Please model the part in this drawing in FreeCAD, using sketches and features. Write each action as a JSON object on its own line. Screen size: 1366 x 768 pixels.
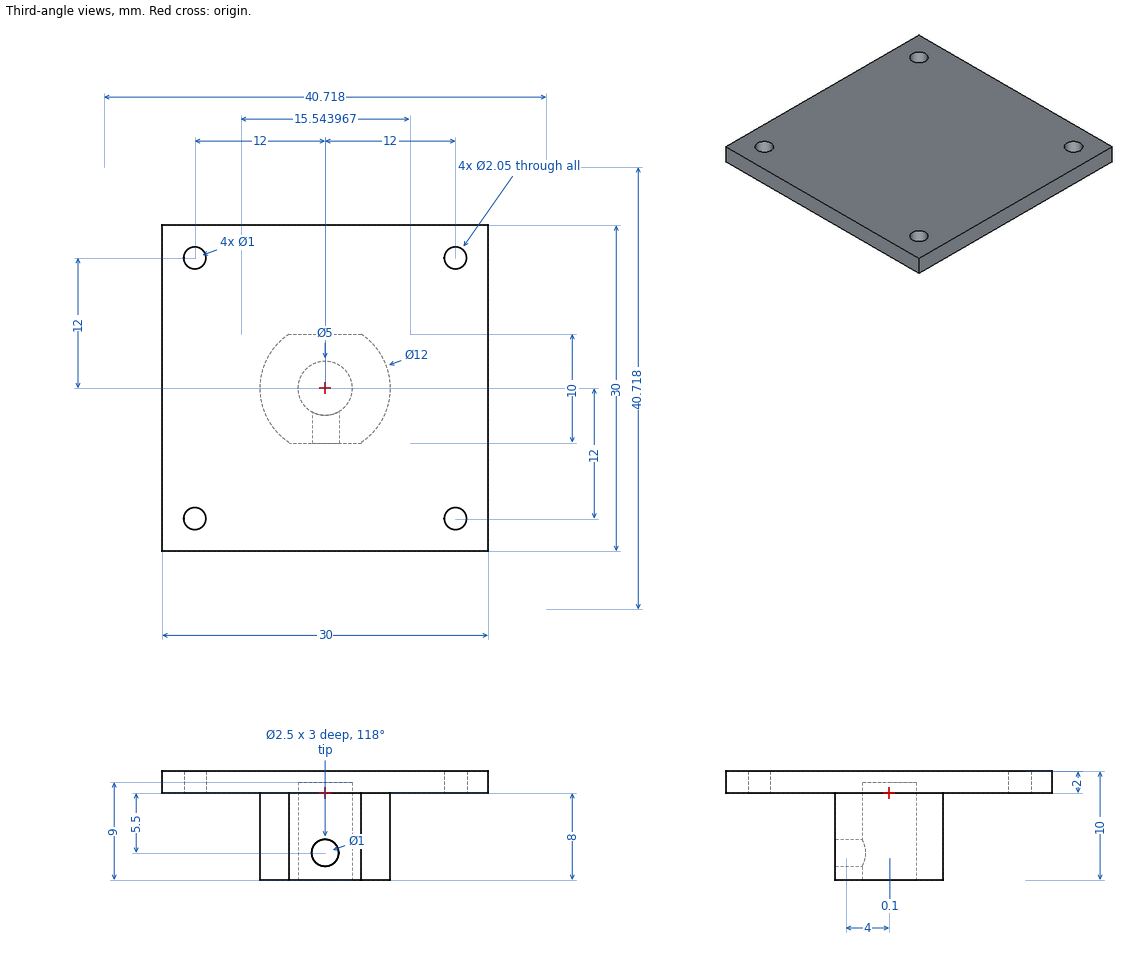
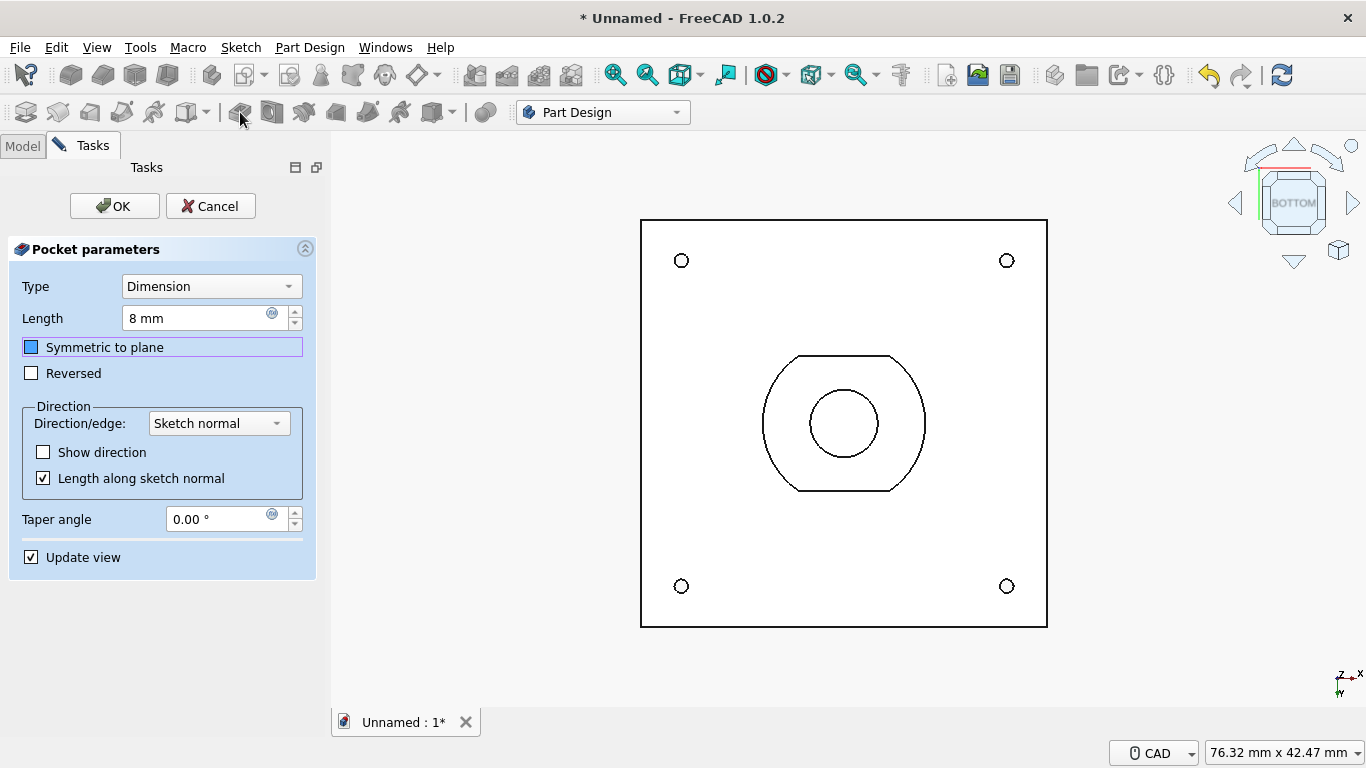
{"action": "left_click", "coordinate": [115, 206]}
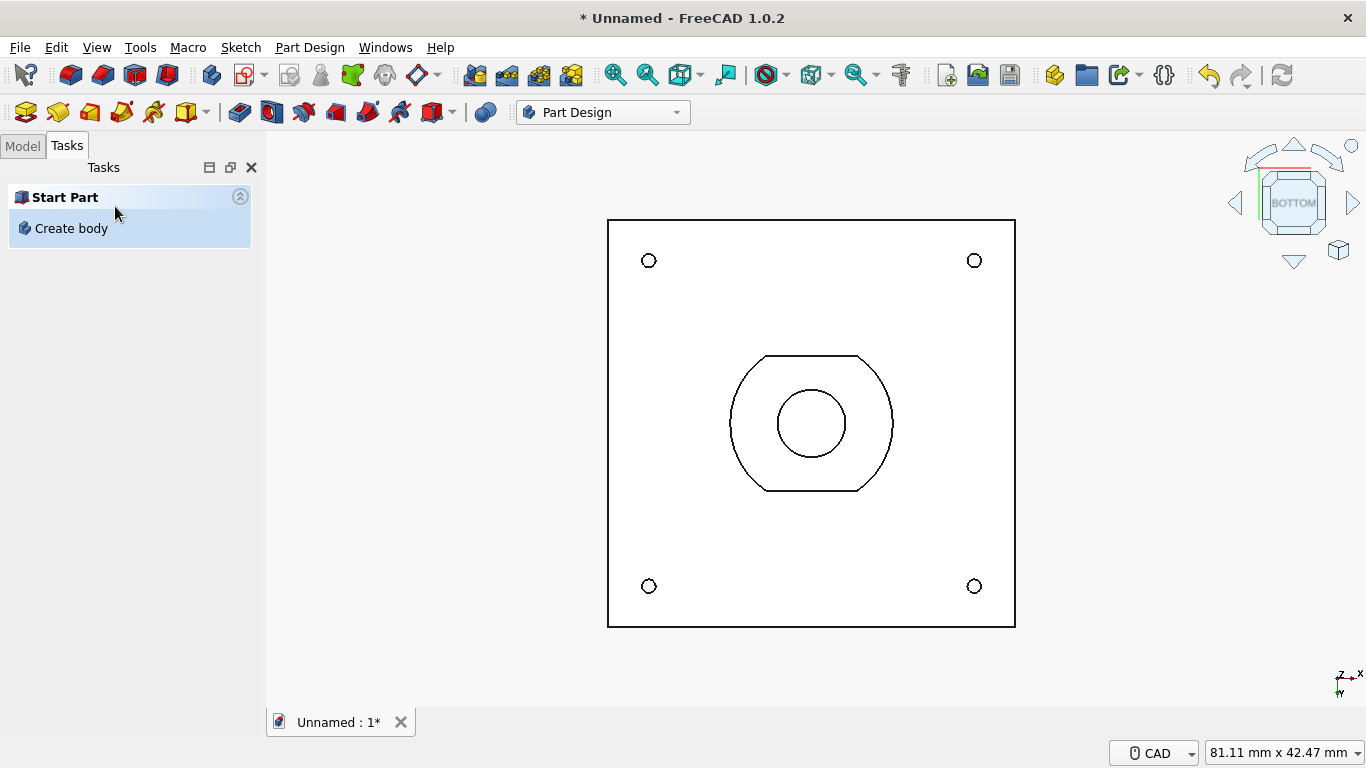
{"action": "key", "text": "0"}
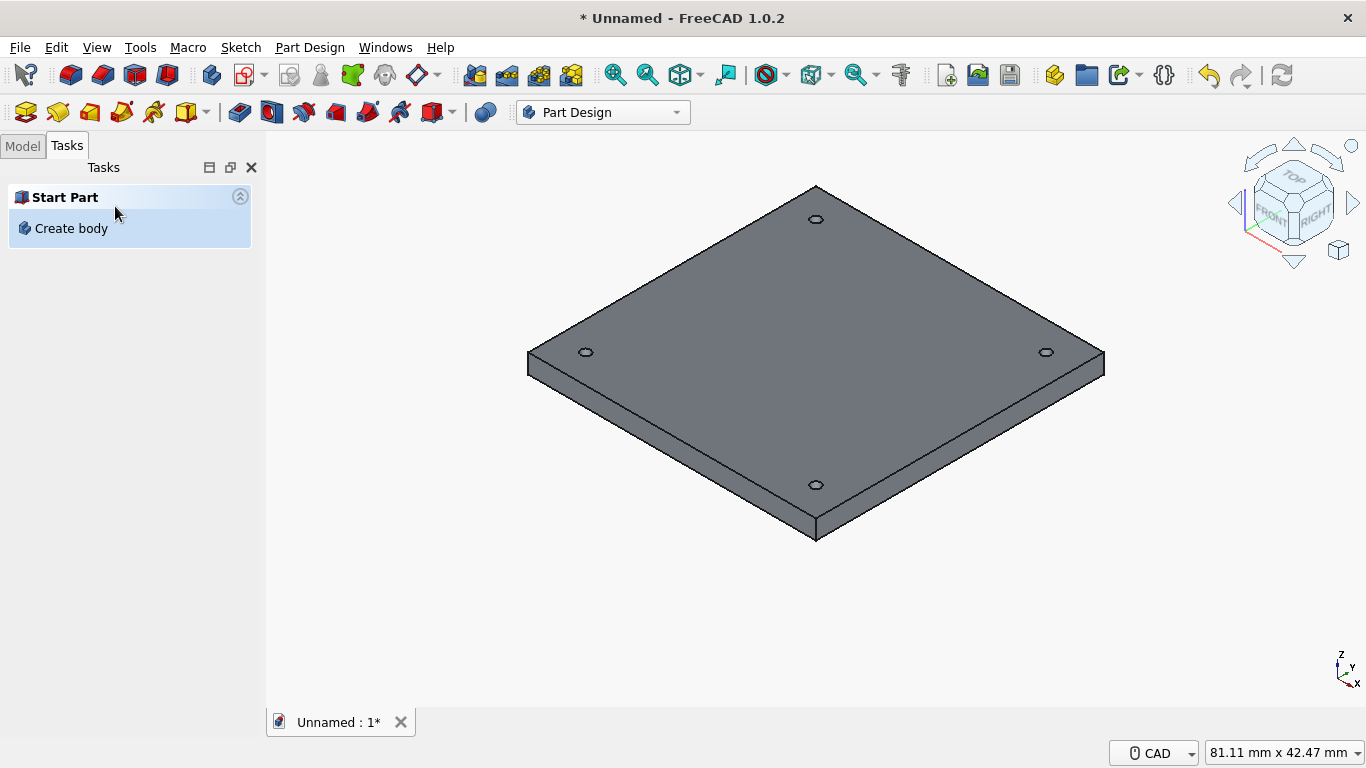
{"action": "key", "text": "1"}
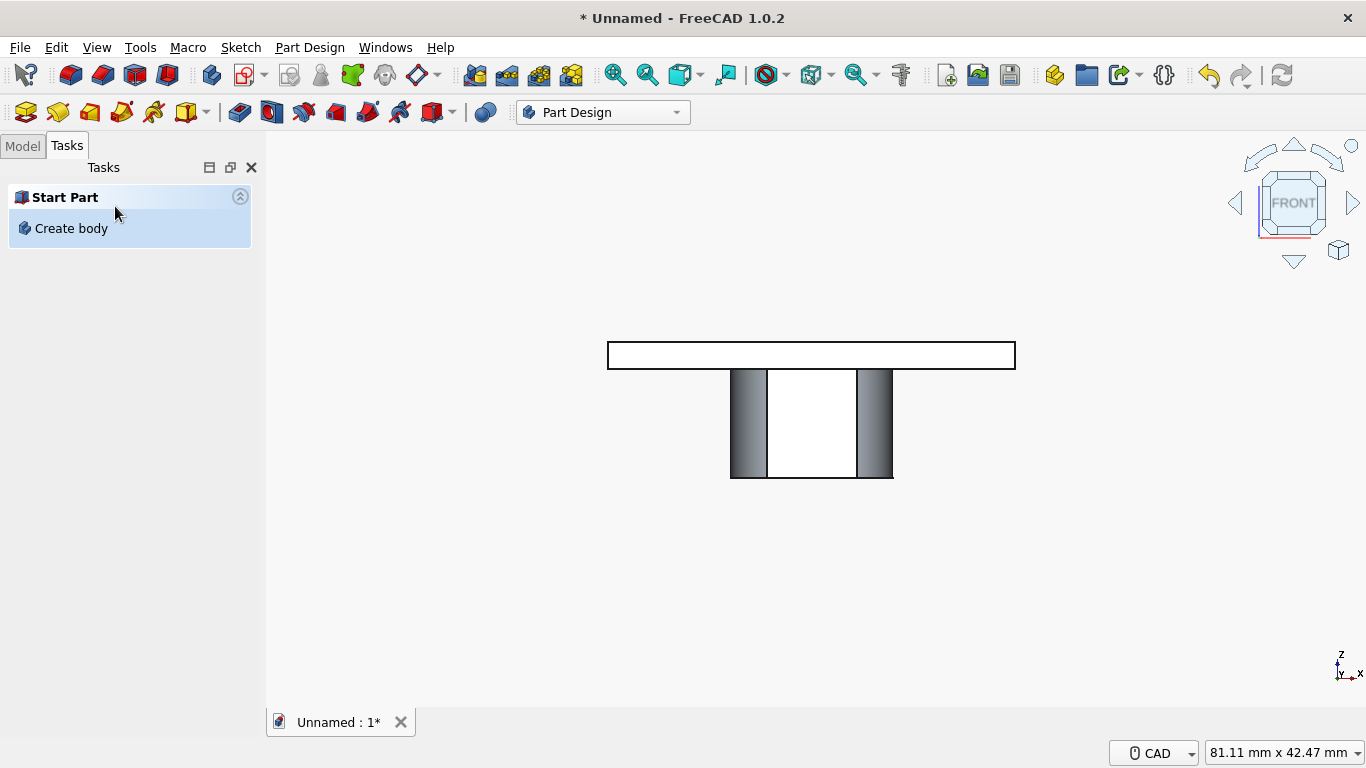
{"action": "left_click", "coordinate": [616, 76]}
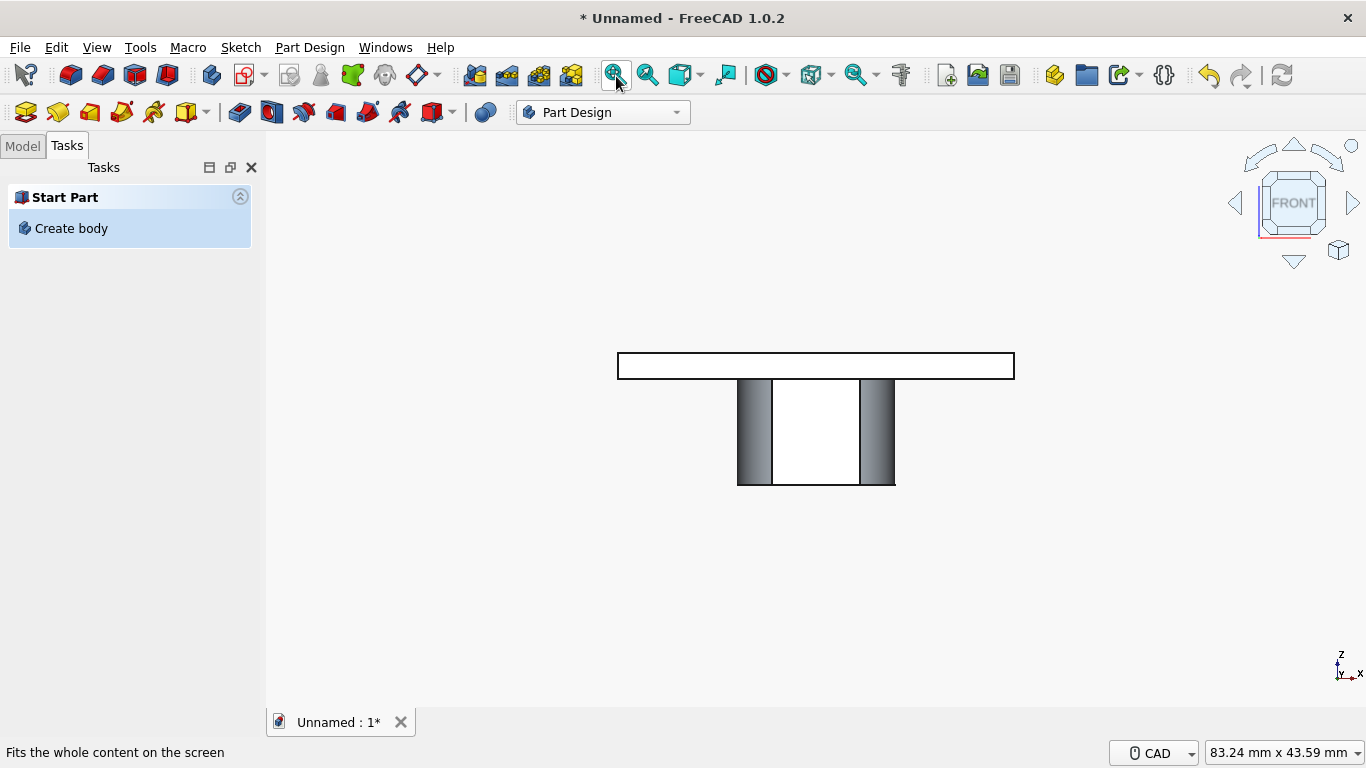
{"action": "left_click", "coordinate": [816, 431]}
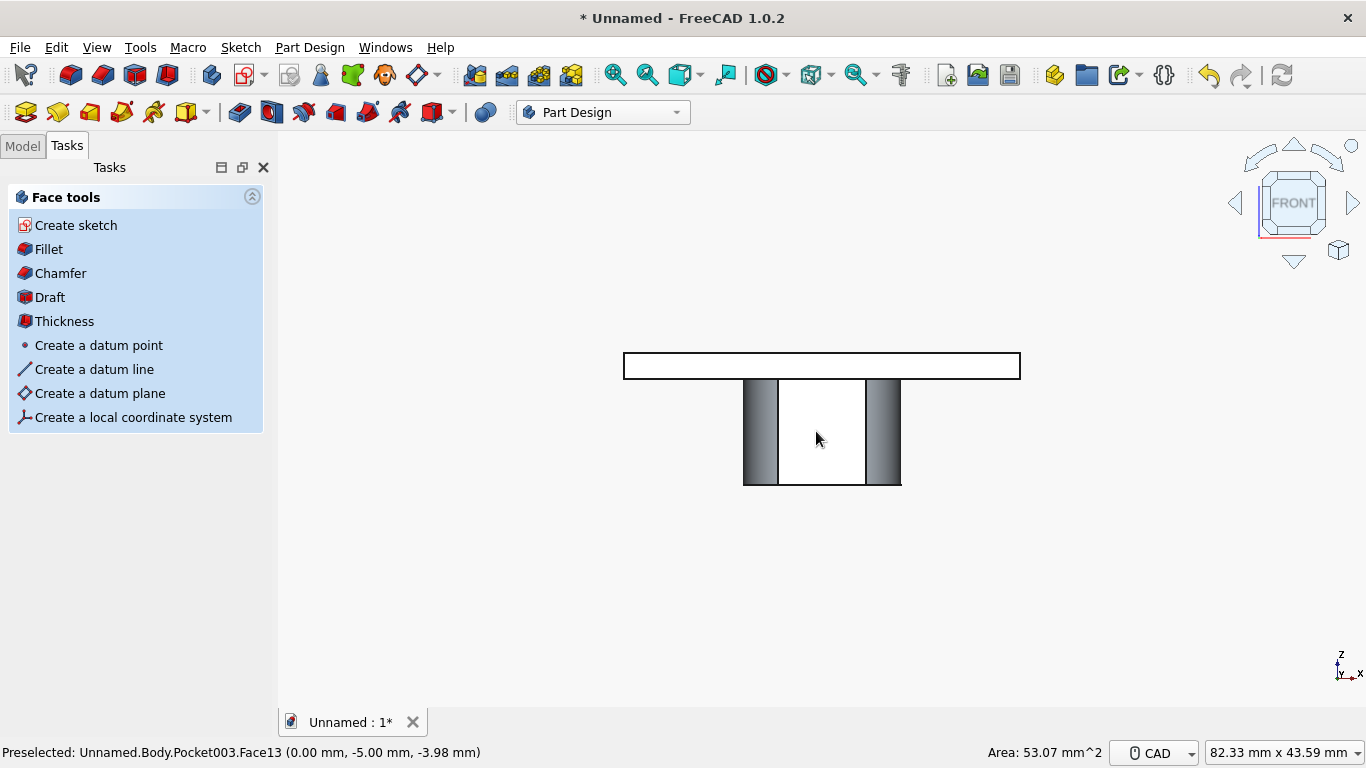
{"action": "left_click", "coordinate": [244, 76]}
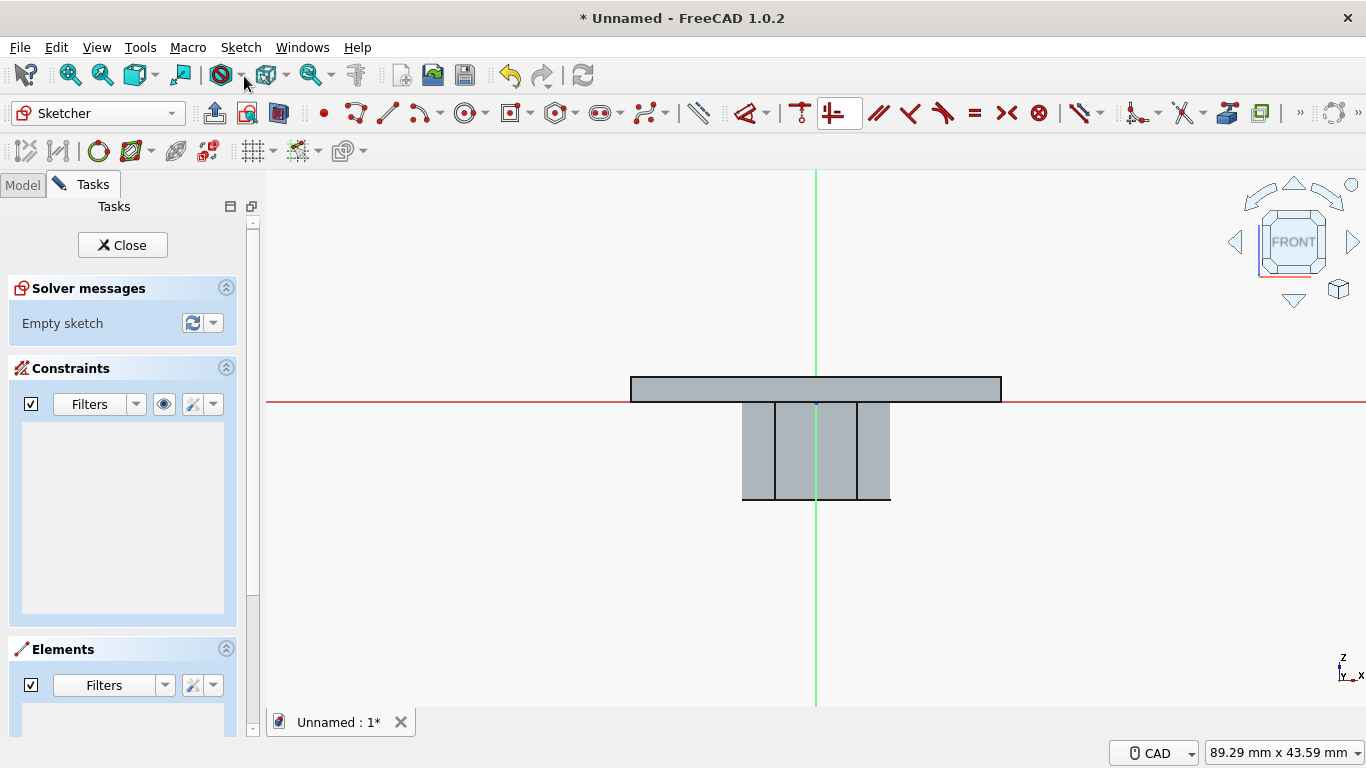
{"action": "scroll", "coordinate": [823, 472], "scroll_direction": "up", "scroll_amount": 12}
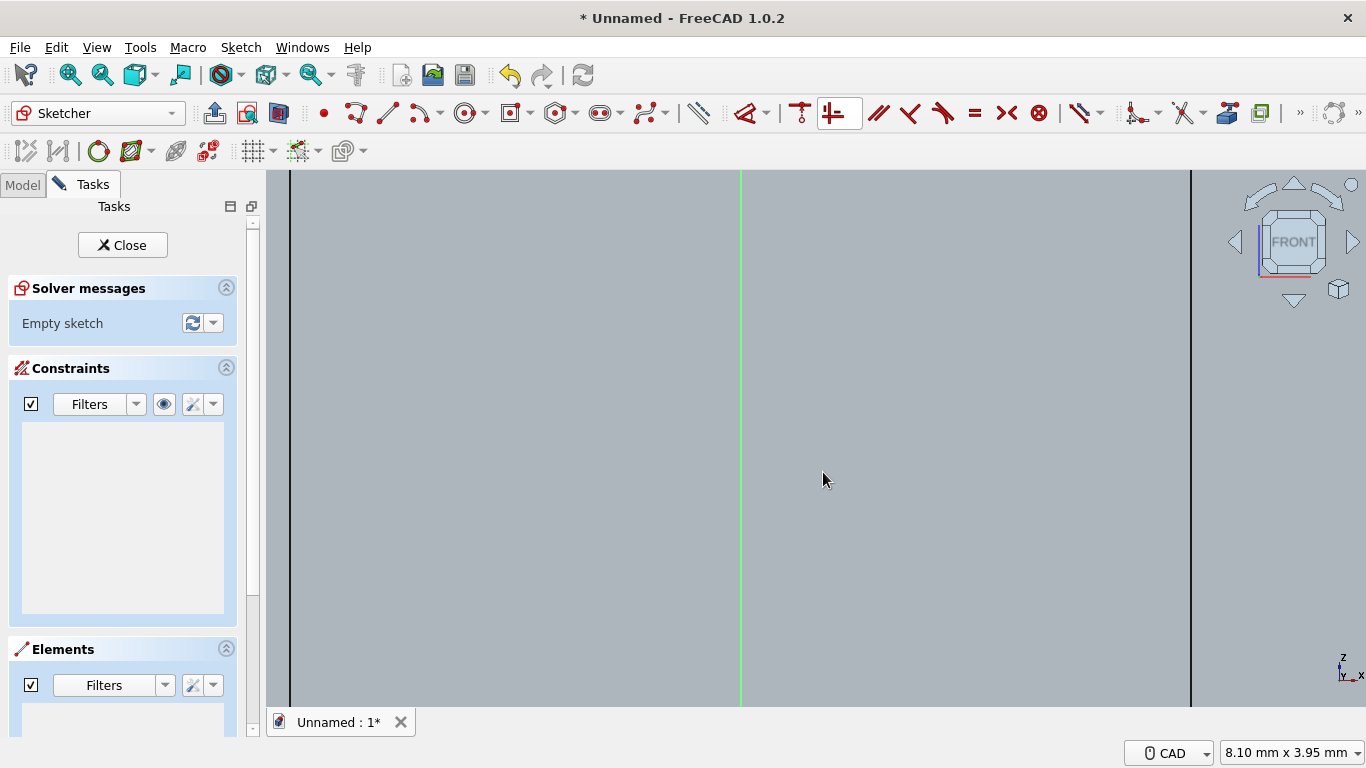
{"action": "key", "text": "g c"}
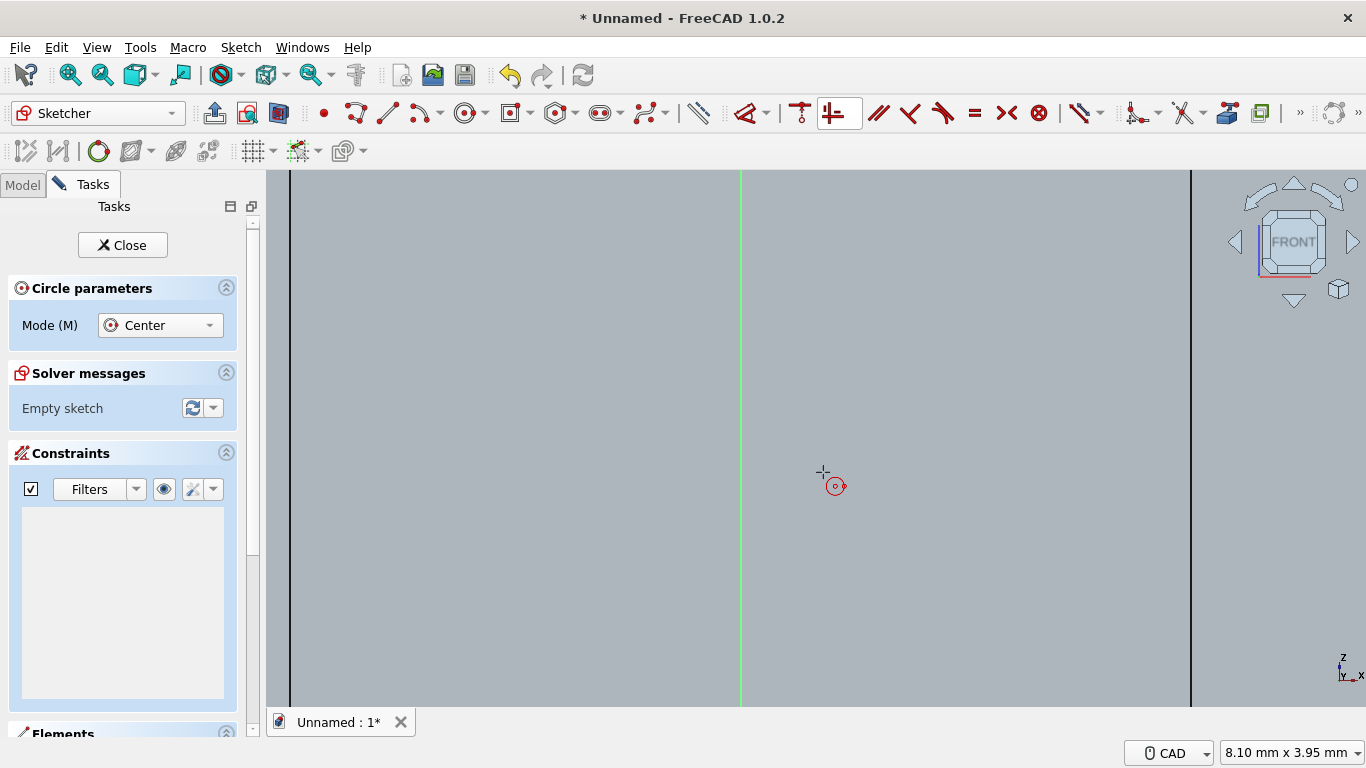
{"action": "left_click", "coordinate": [741, 437]}
{"action": "left_click", "coordinate": [861, 317]}
{"action": "key", "text": "Escape"}